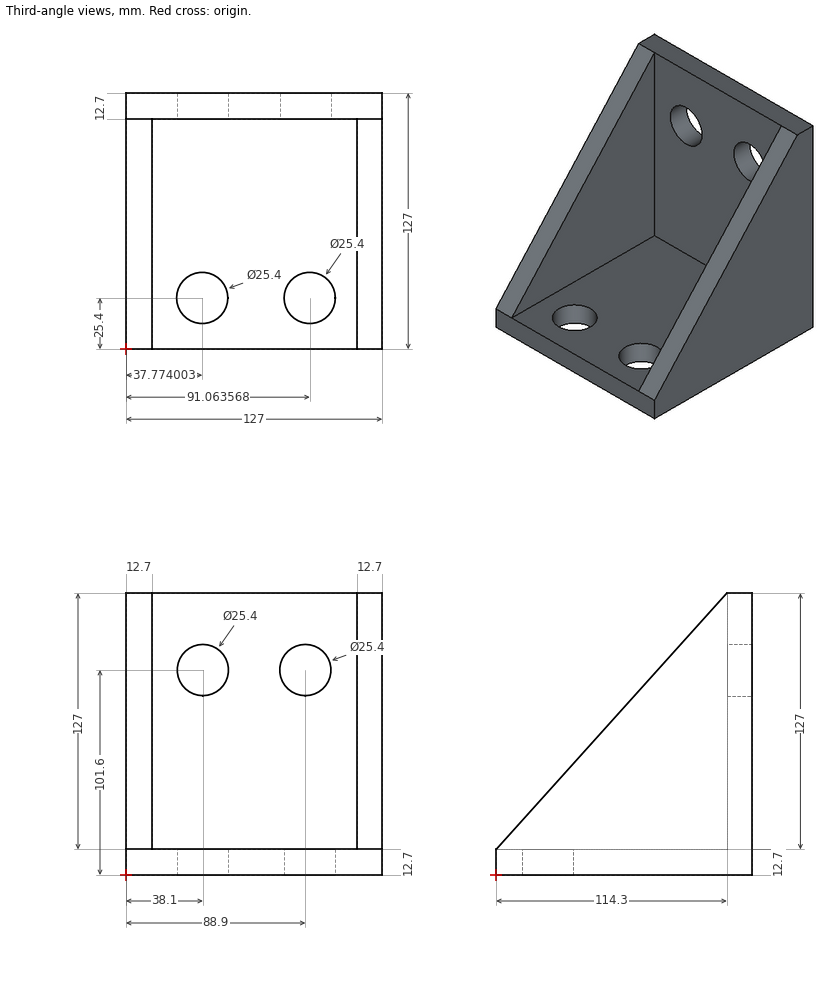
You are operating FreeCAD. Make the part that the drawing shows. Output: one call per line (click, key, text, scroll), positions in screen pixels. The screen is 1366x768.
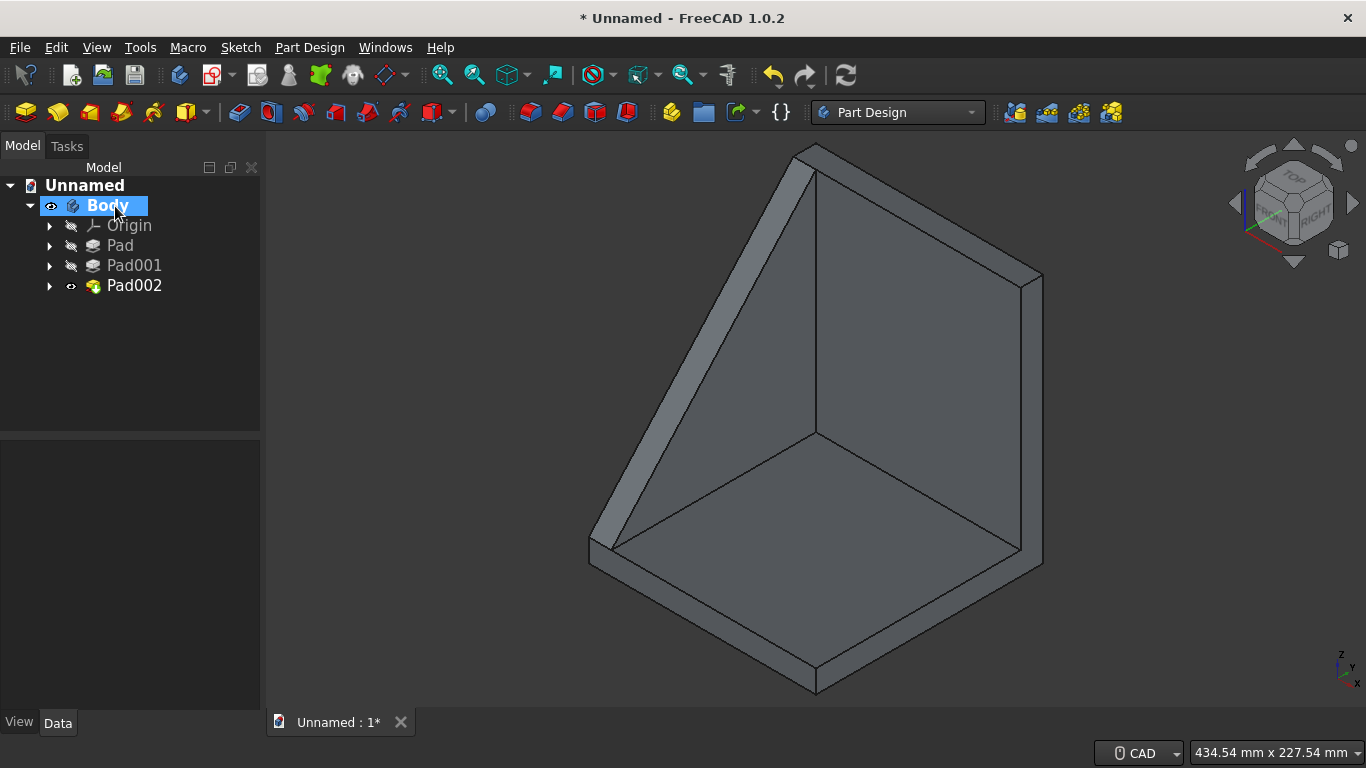
key(3)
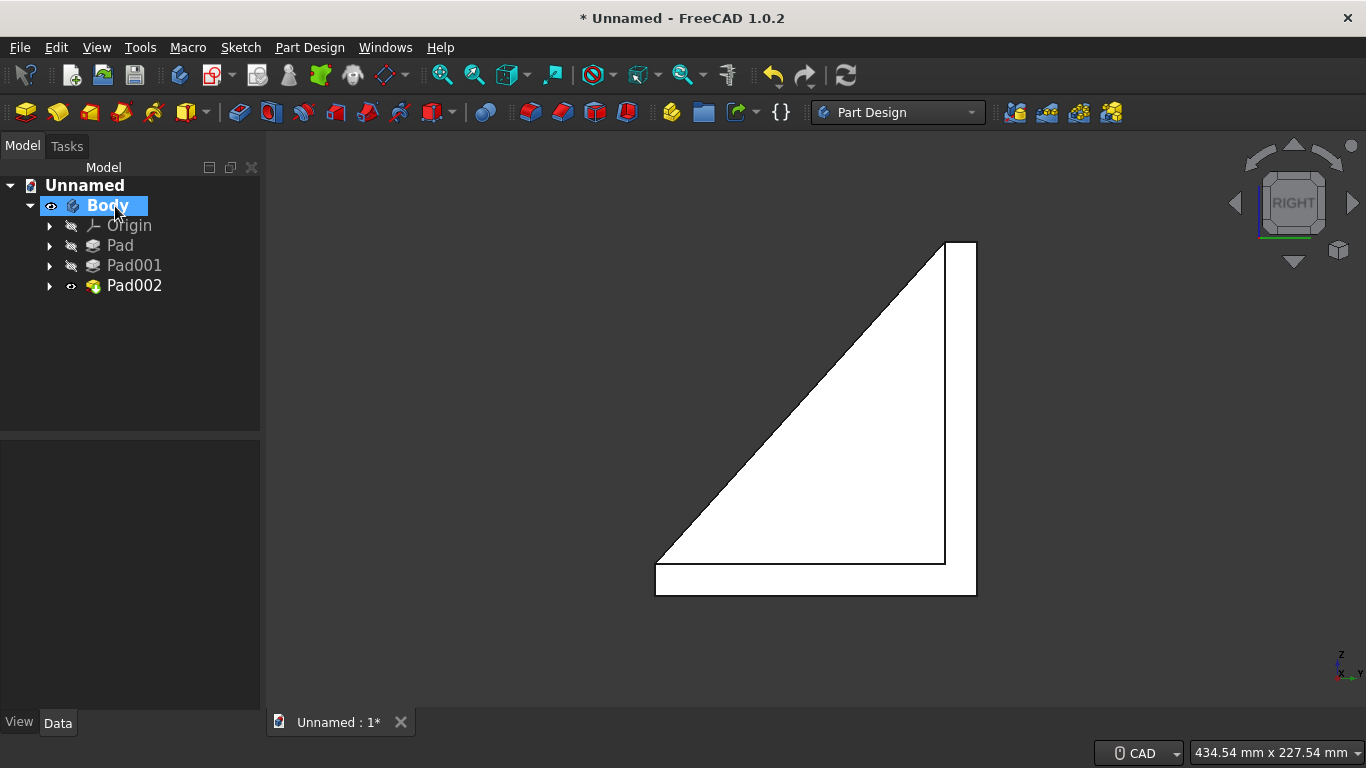
click(954, 570)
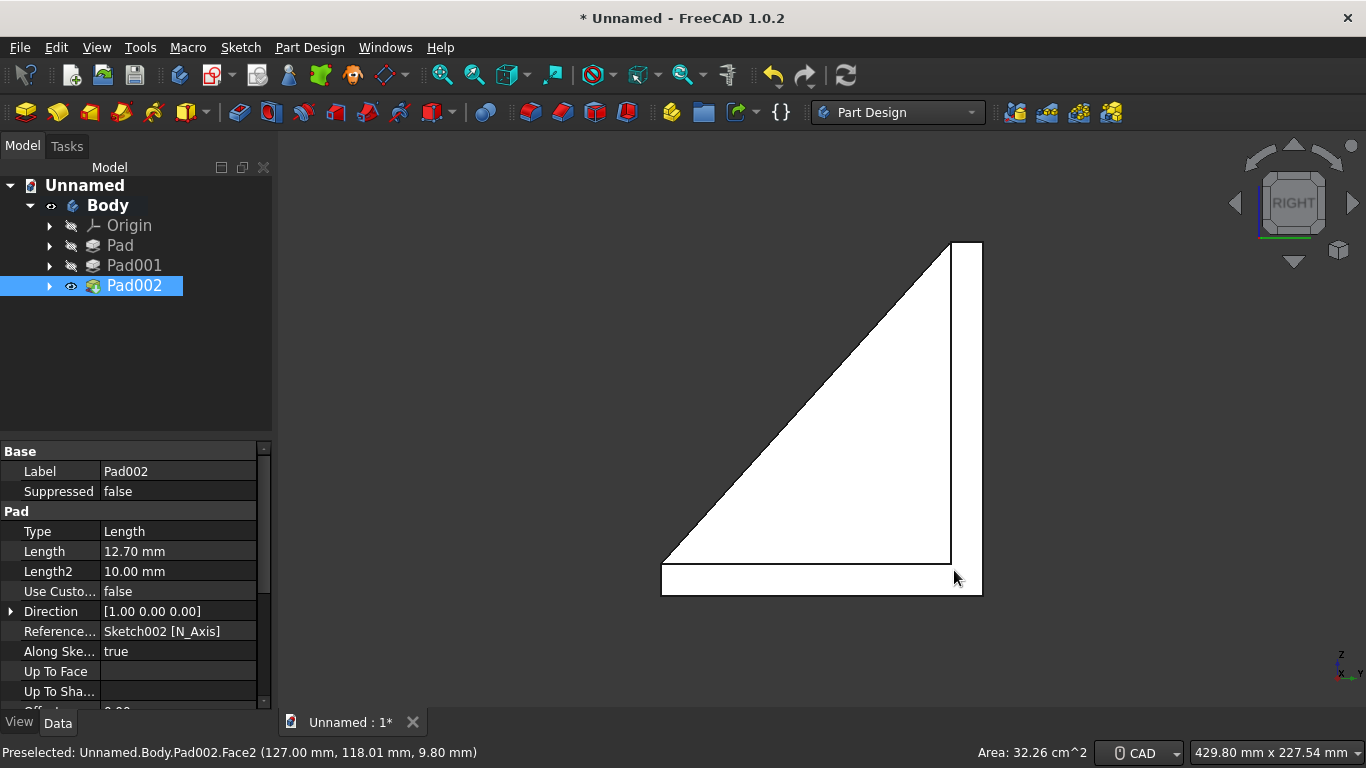
click(212, 76)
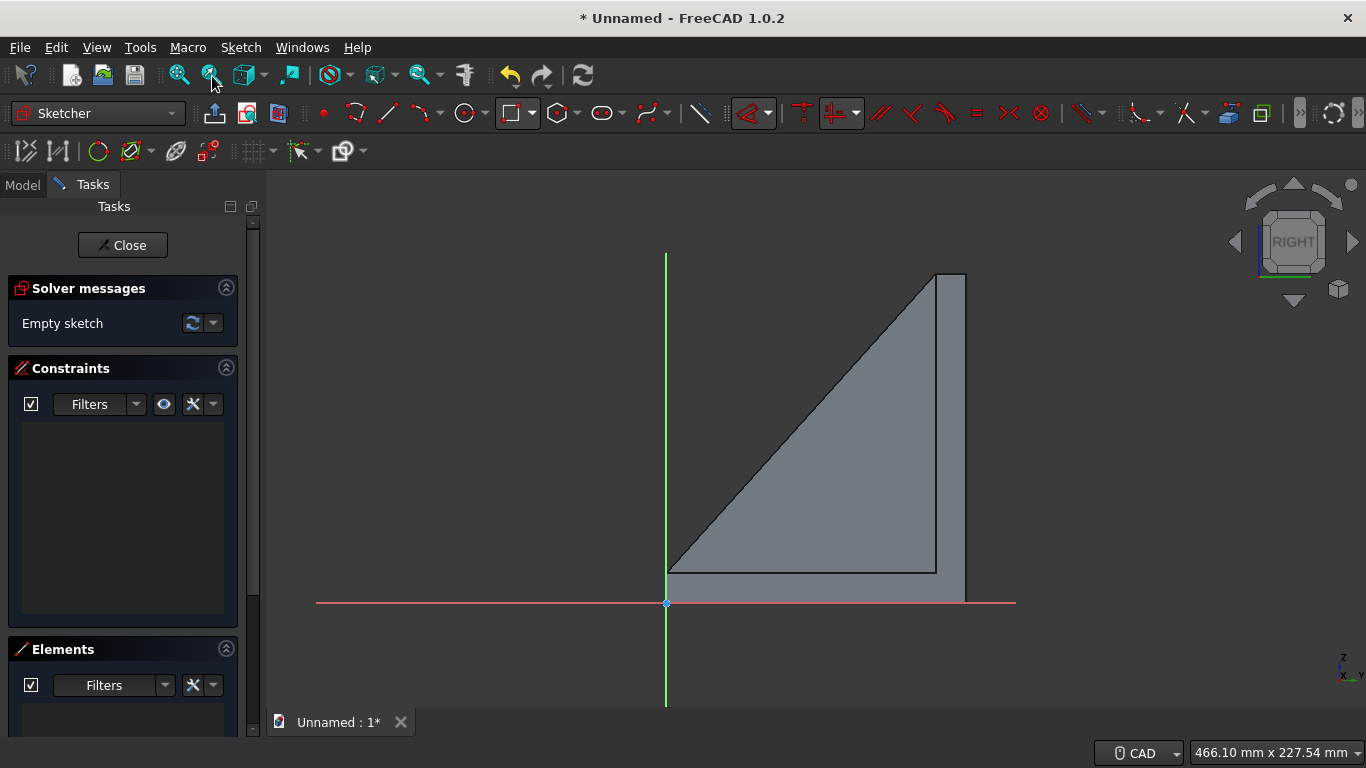
click(356, 114)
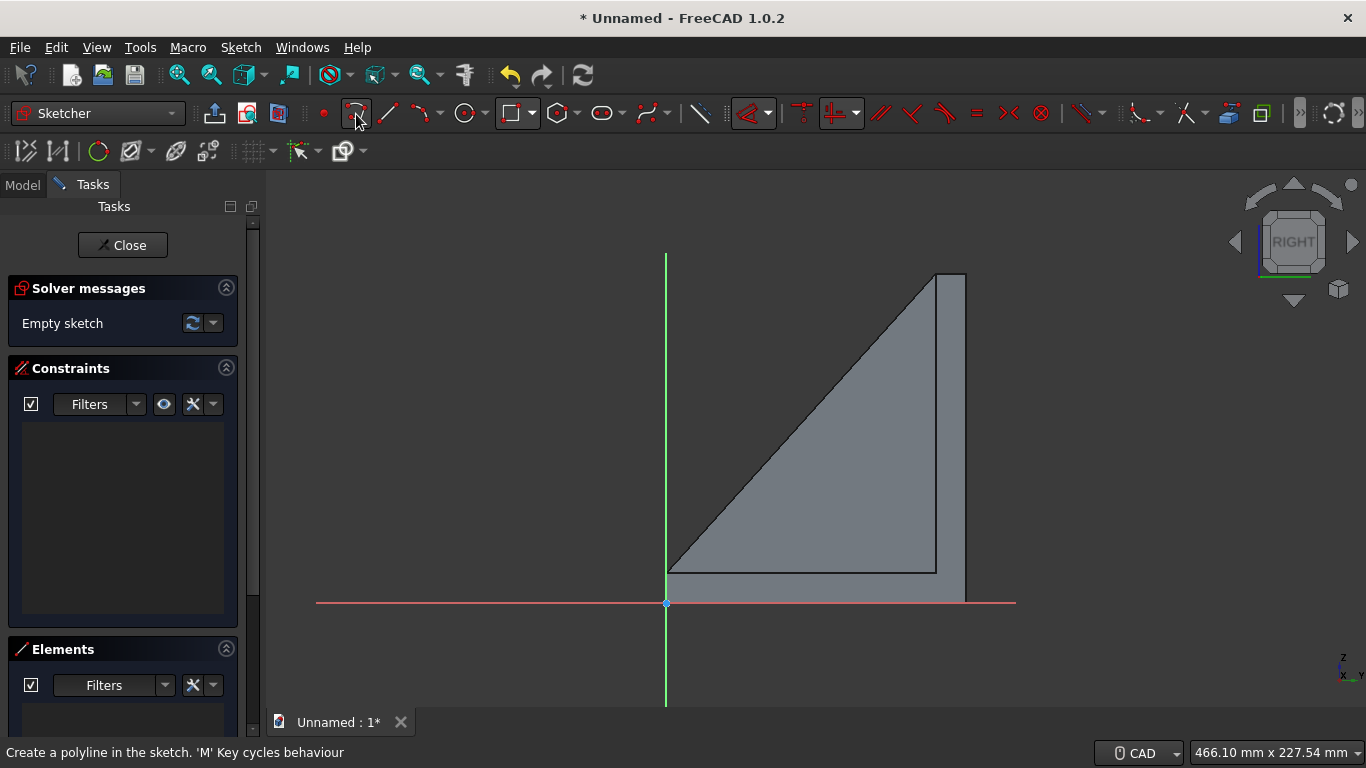
click(666, 573)
click(936, 573)
click(936, 274)
click(666, 574)
key(Escape)
key(Escape)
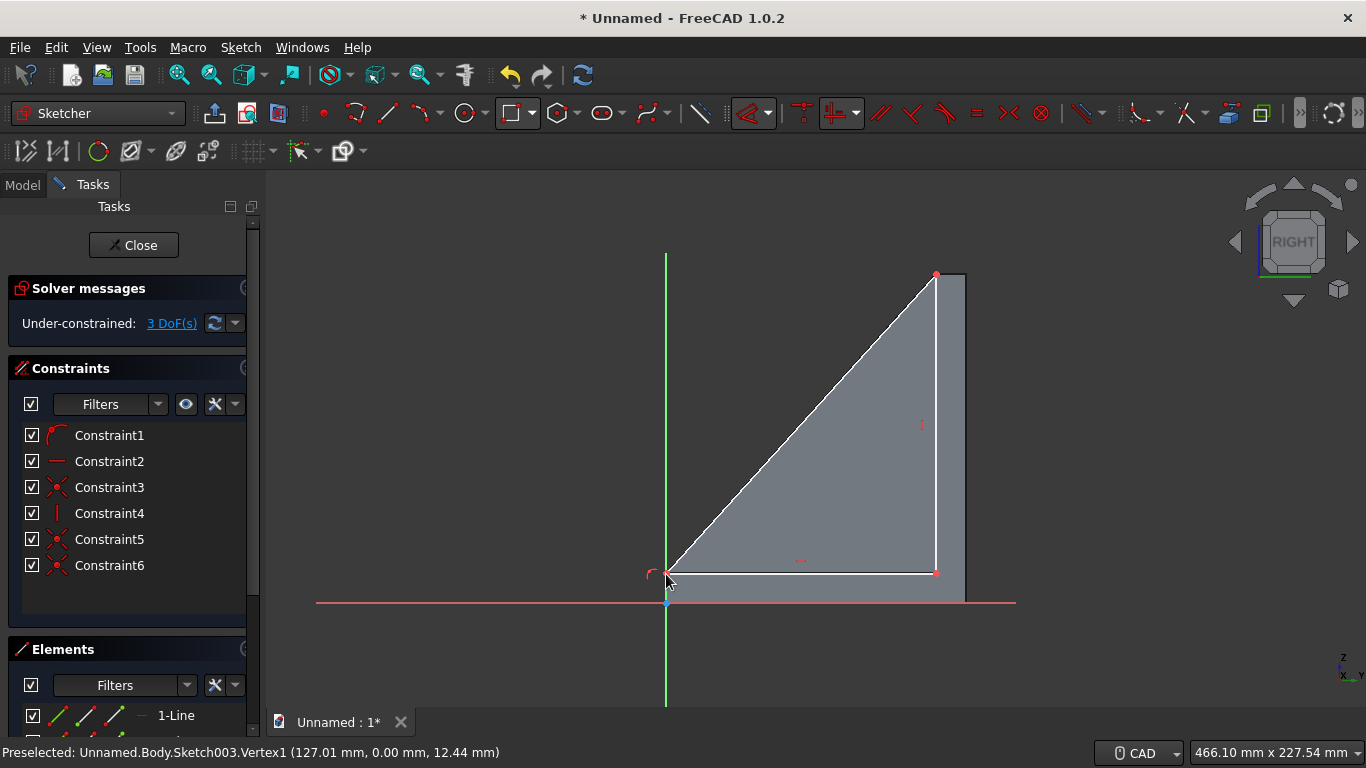
click(936, 484)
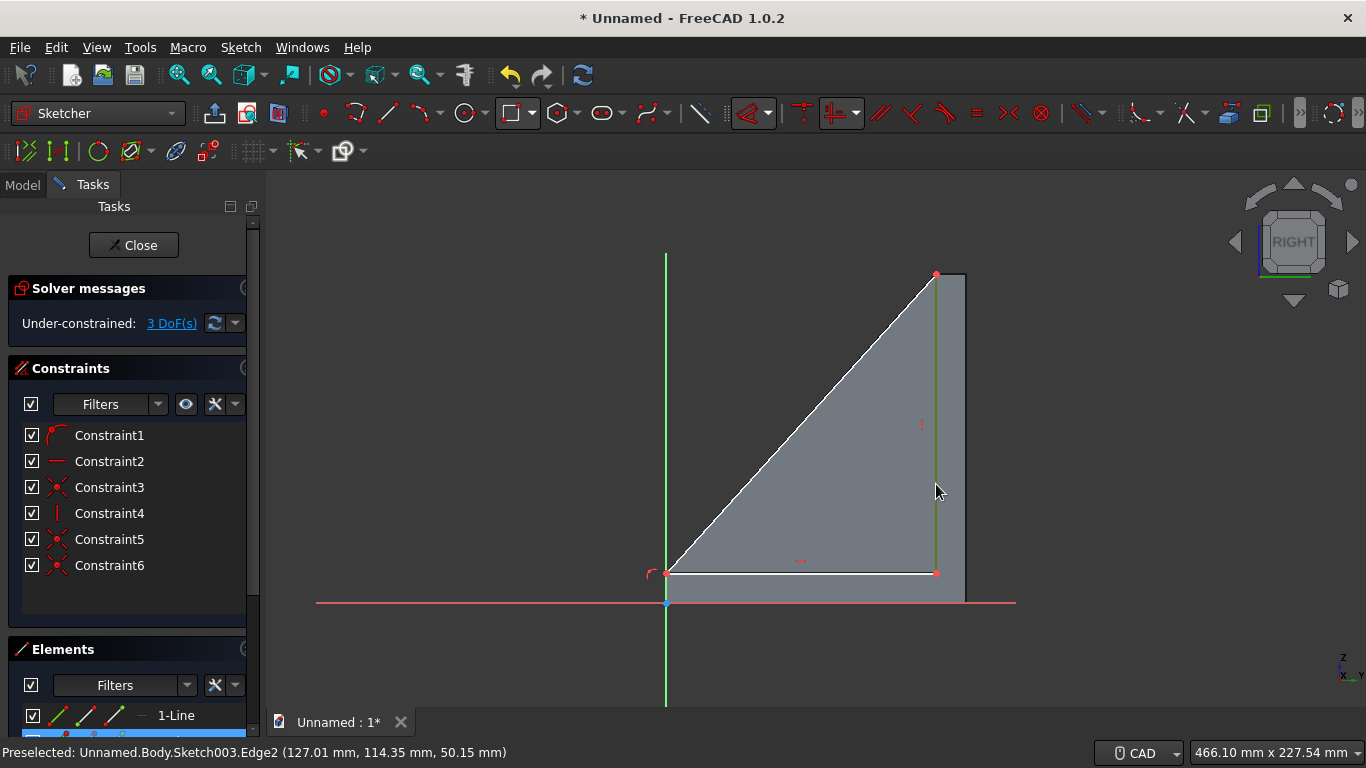
key(i)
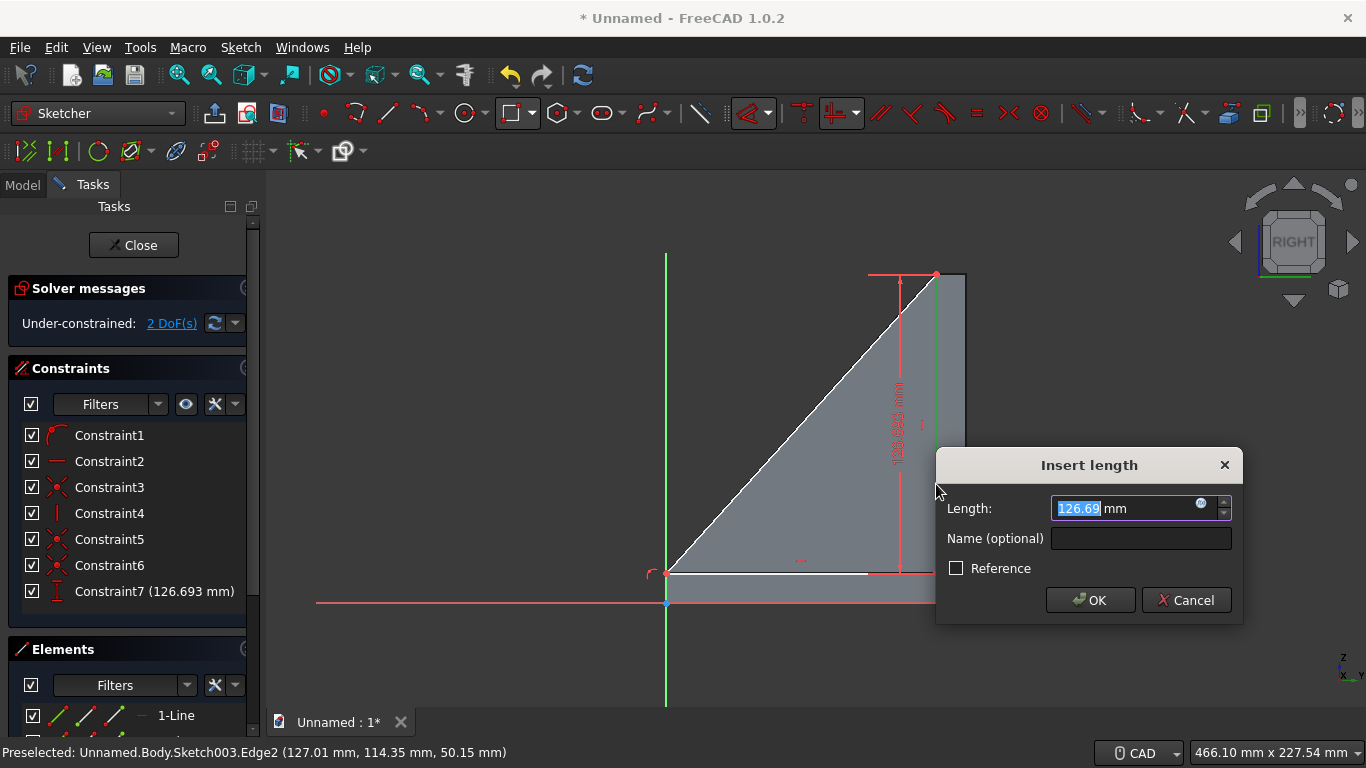
text(127)
key(Return)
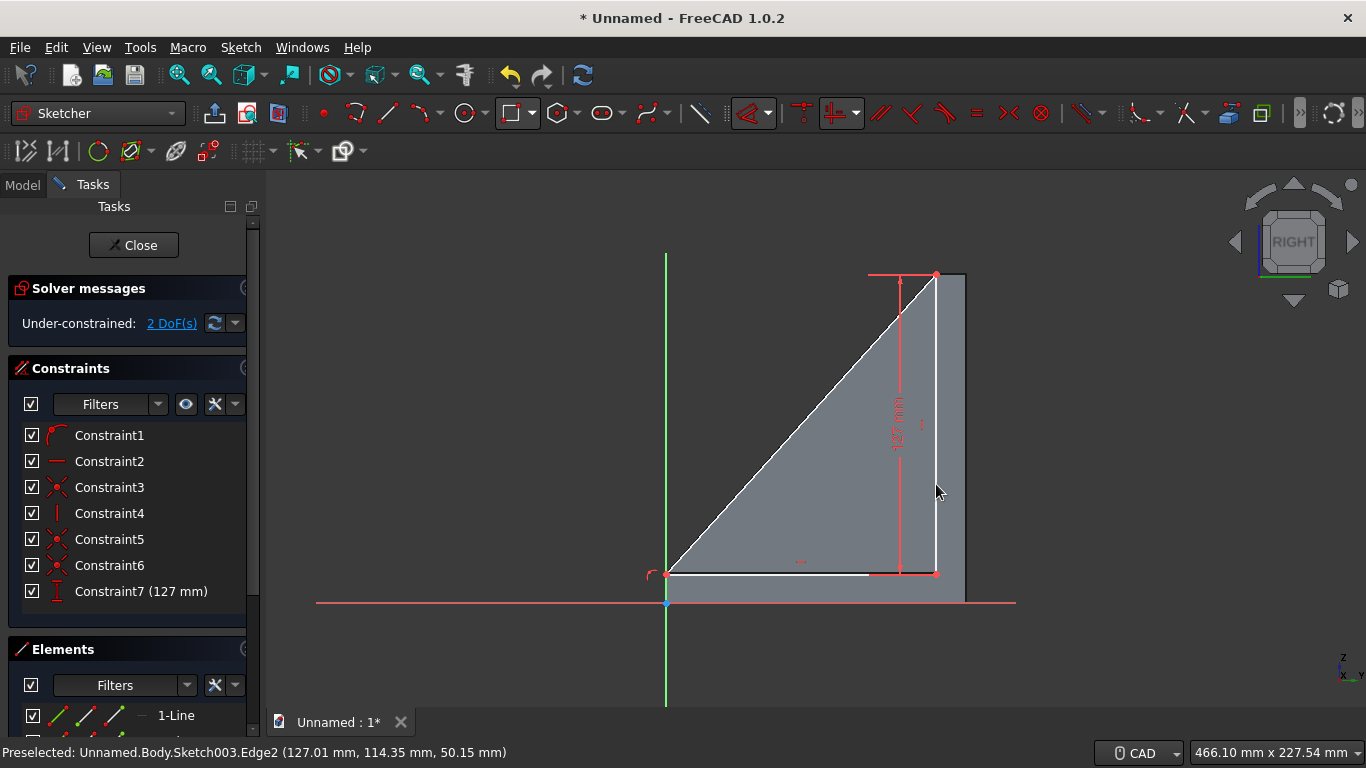
click(747, 575)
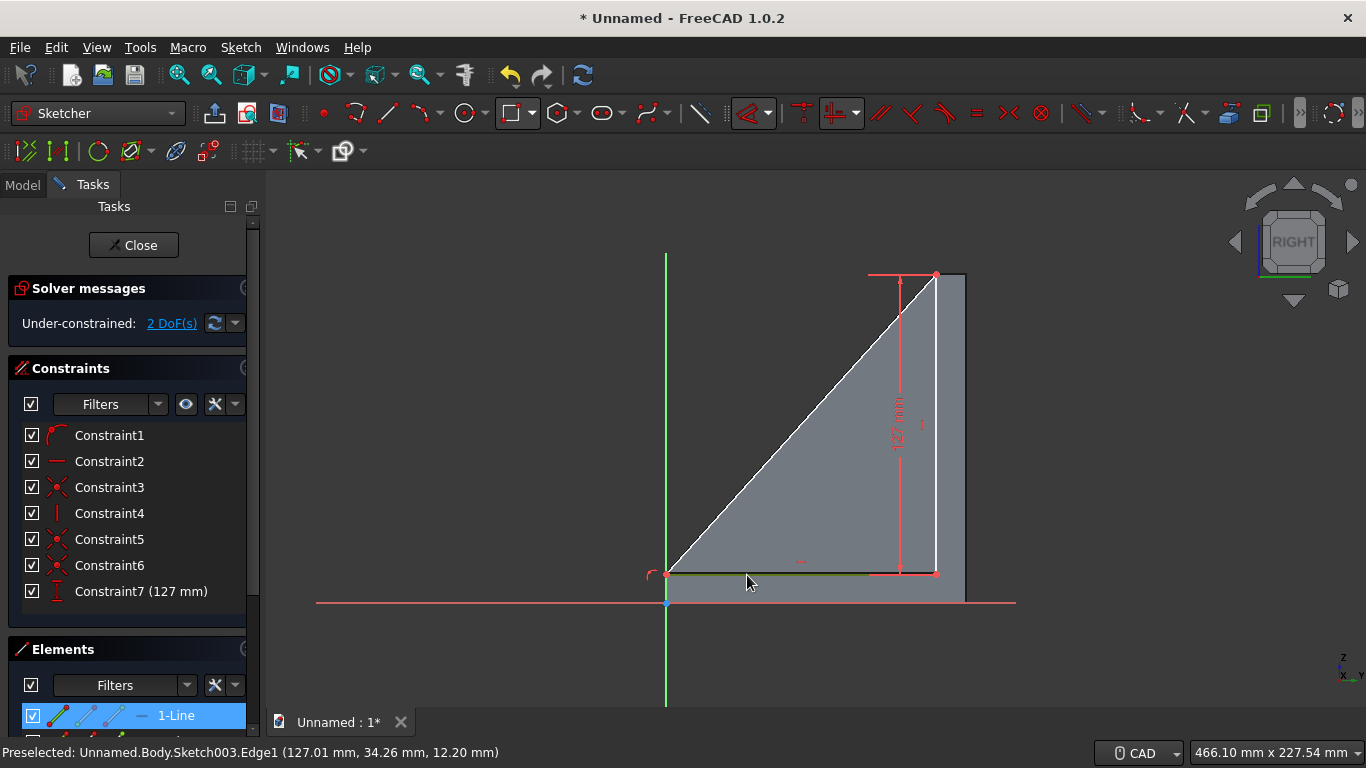
key(l)